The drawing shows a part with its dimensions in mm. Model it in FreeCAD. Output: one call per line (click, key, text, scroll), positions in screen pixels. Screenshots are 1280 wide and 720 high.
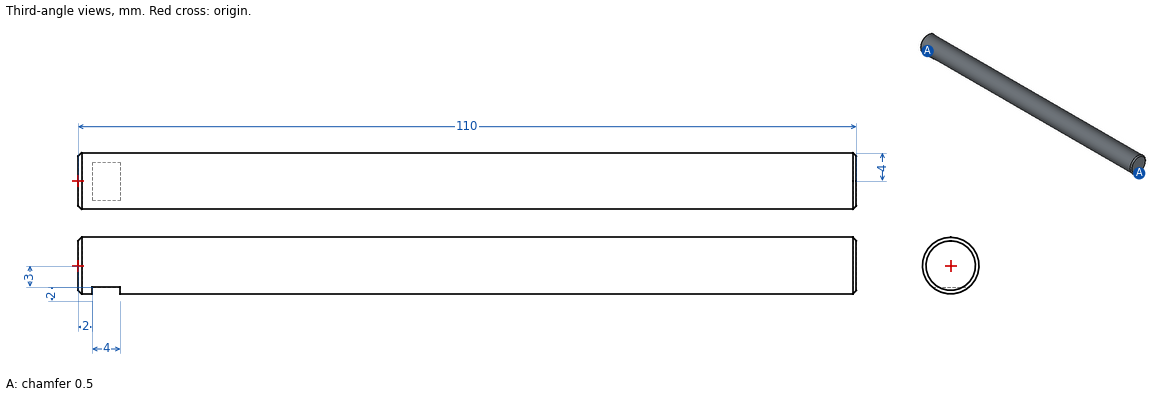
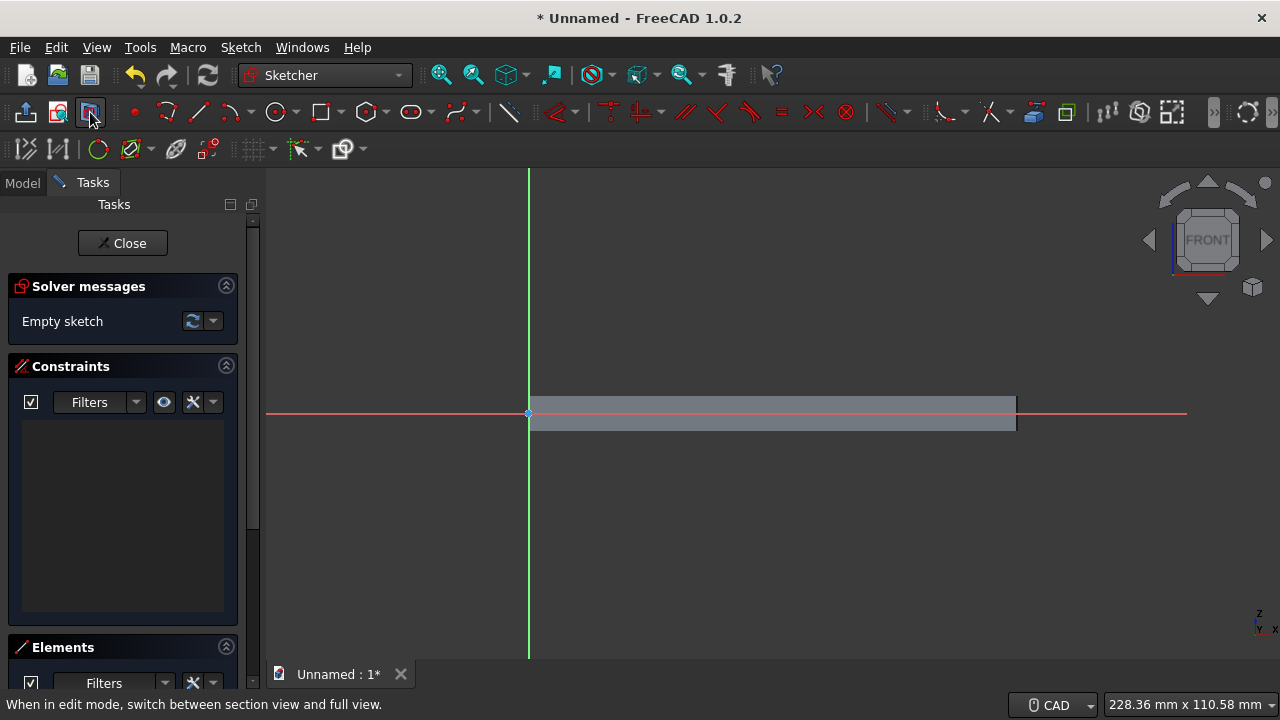
scroll(529, 425, up, 13)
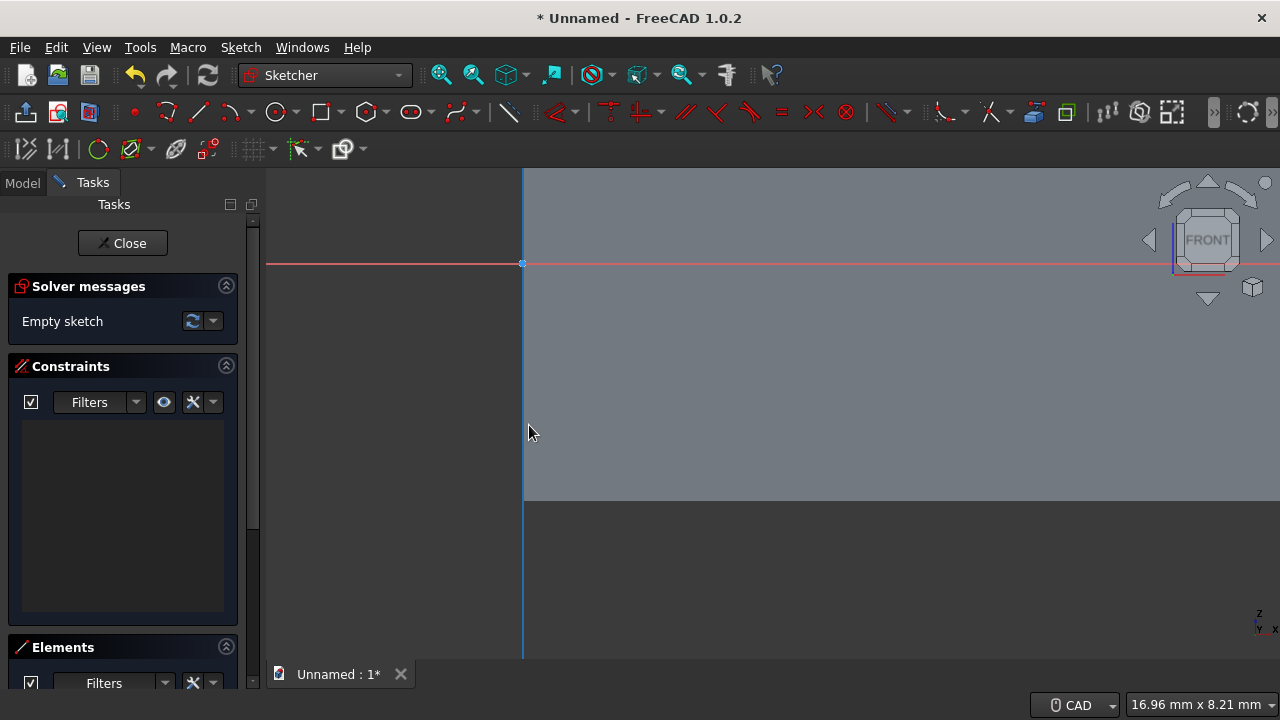
click(322, 112)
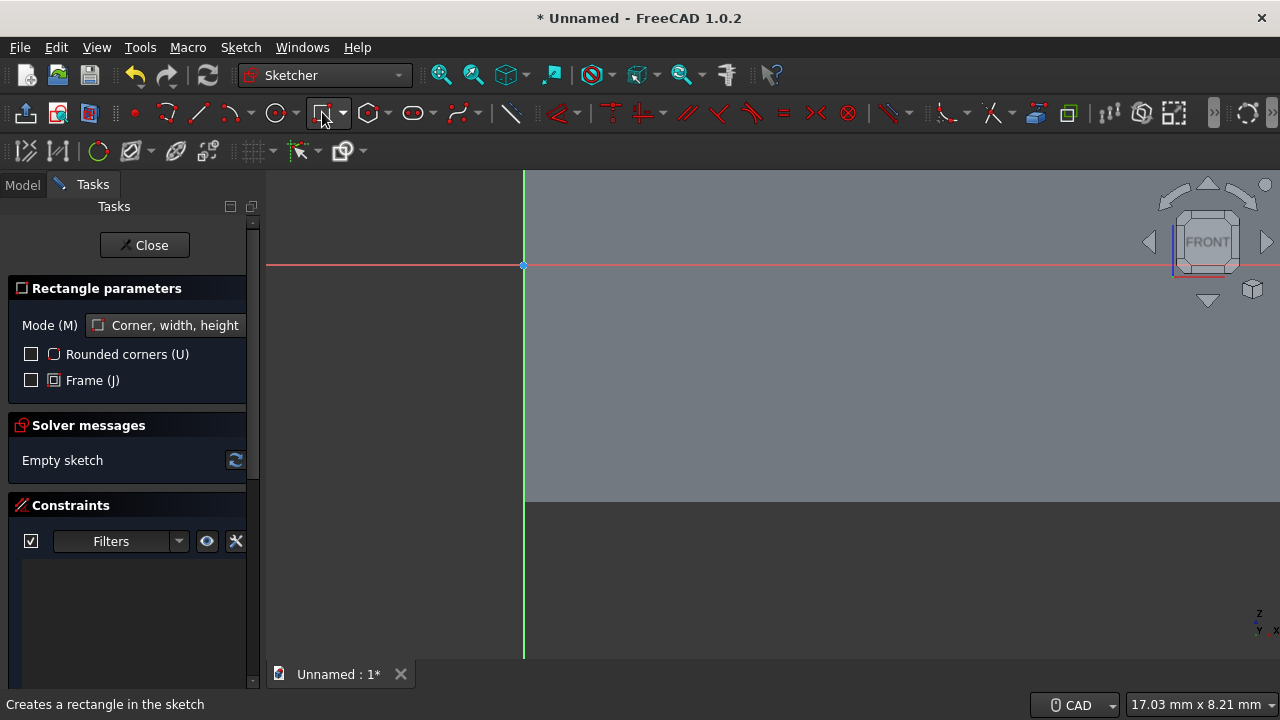
click(643, 444)
click(881, 563)
key(Escape)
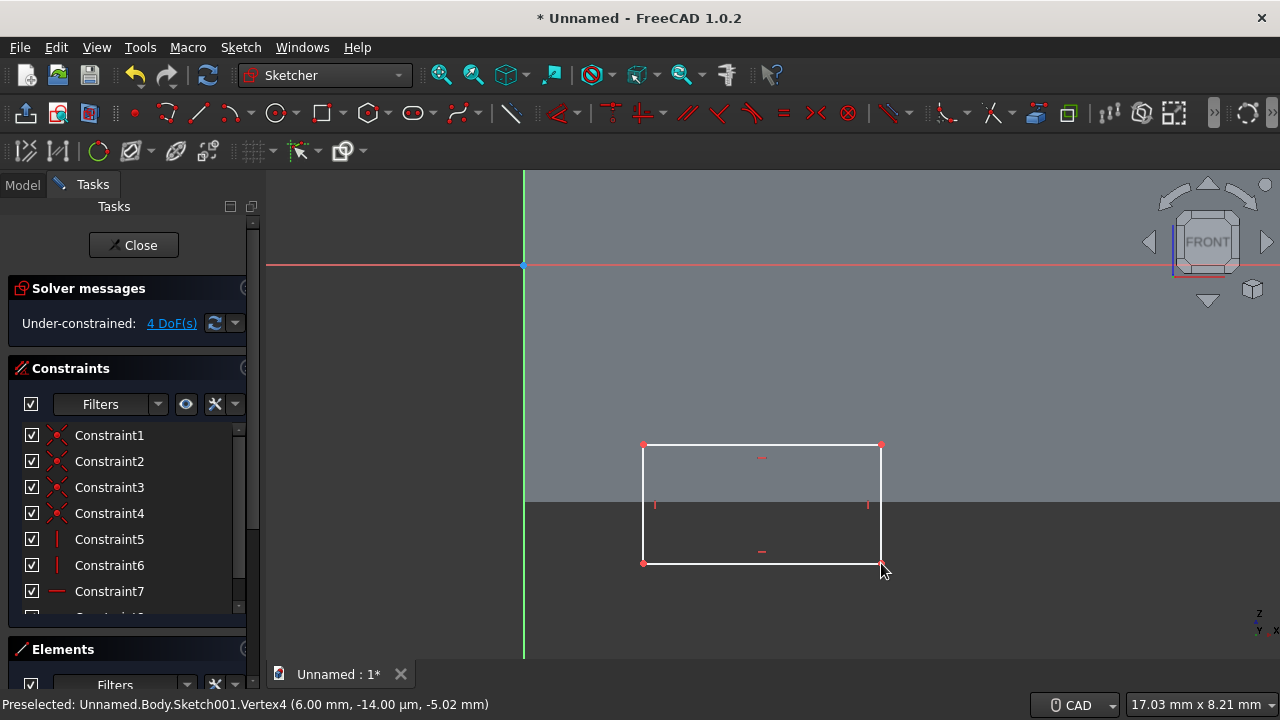
click(558, 114)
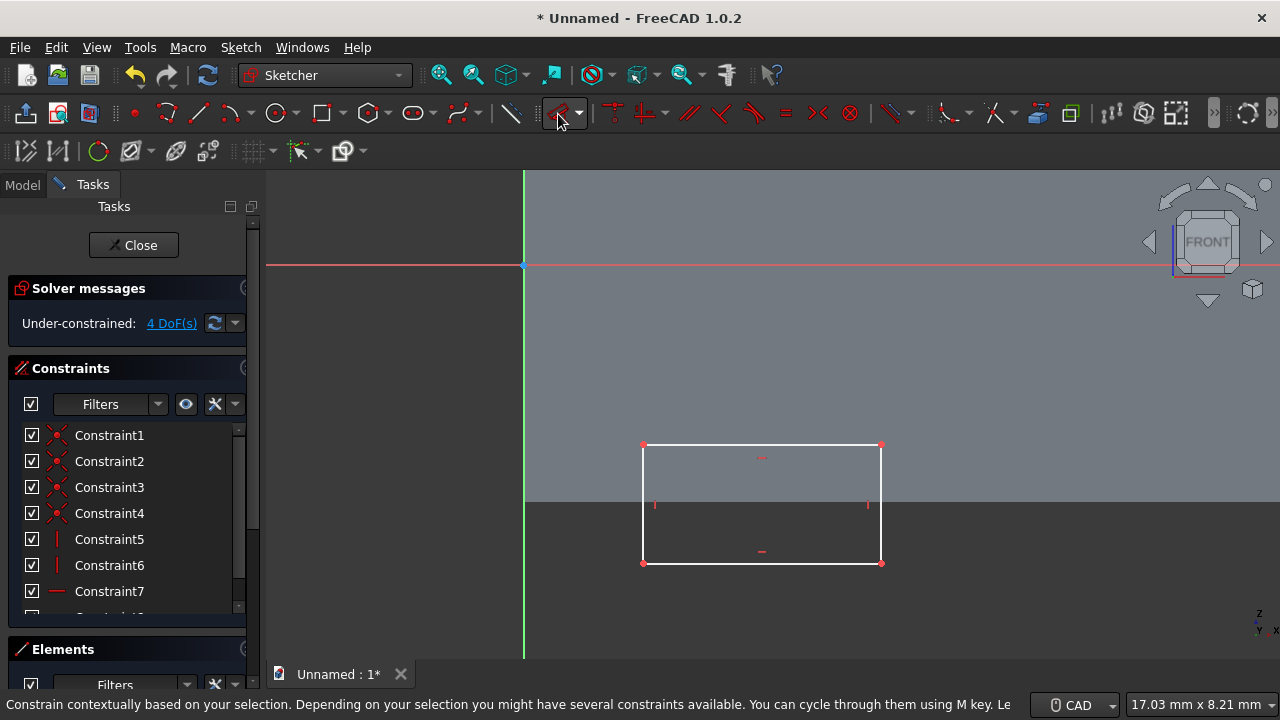
click(643, 481)
click(609, 504)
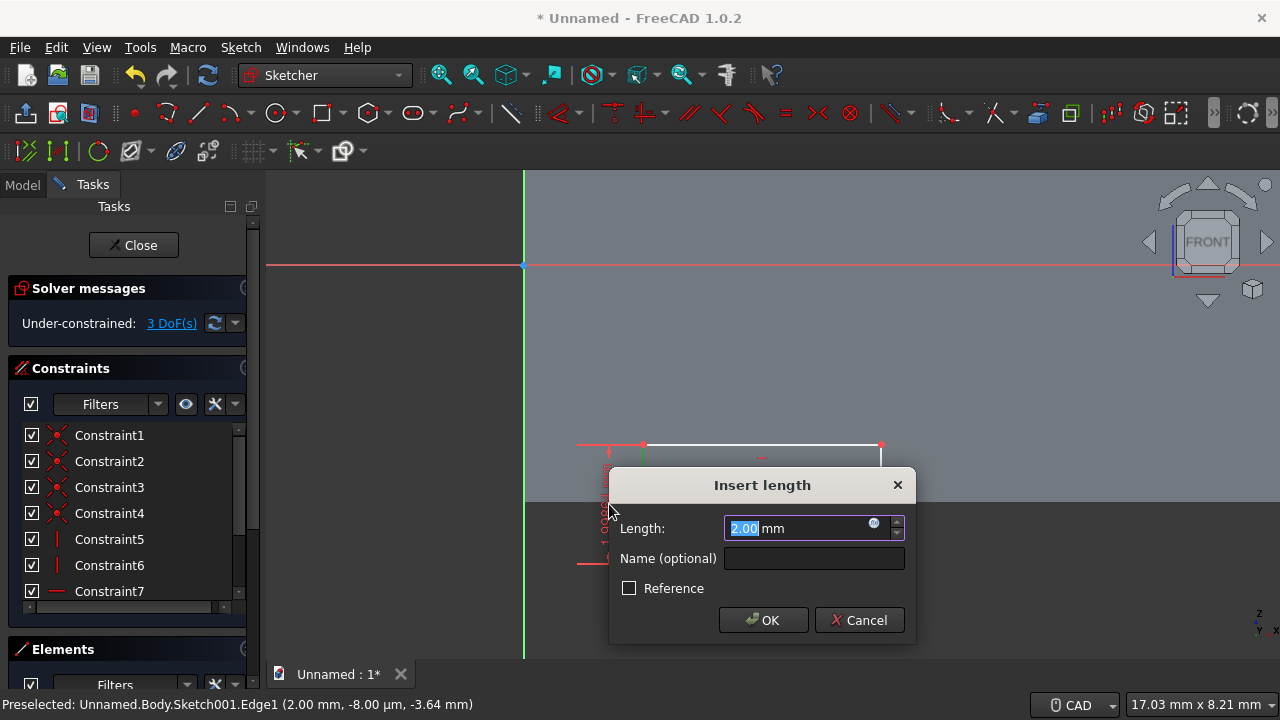
text(2)
key(Return)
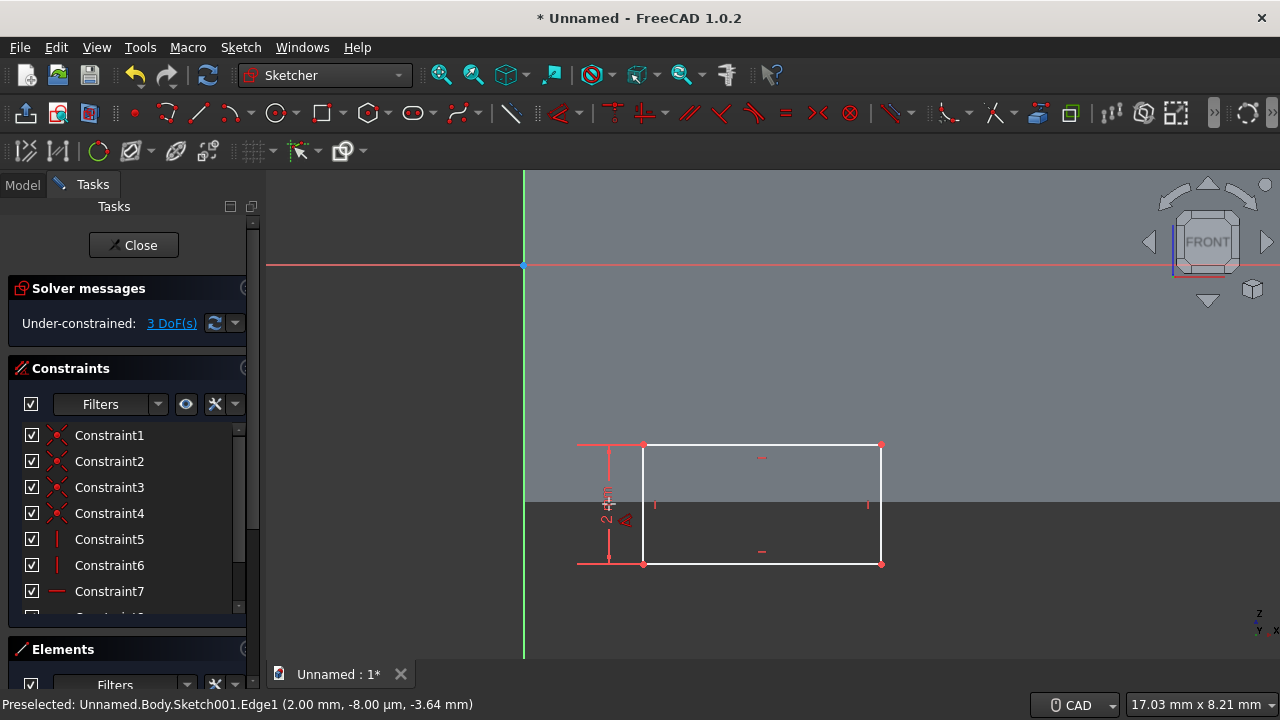
click(714, 564)
click(762, 598)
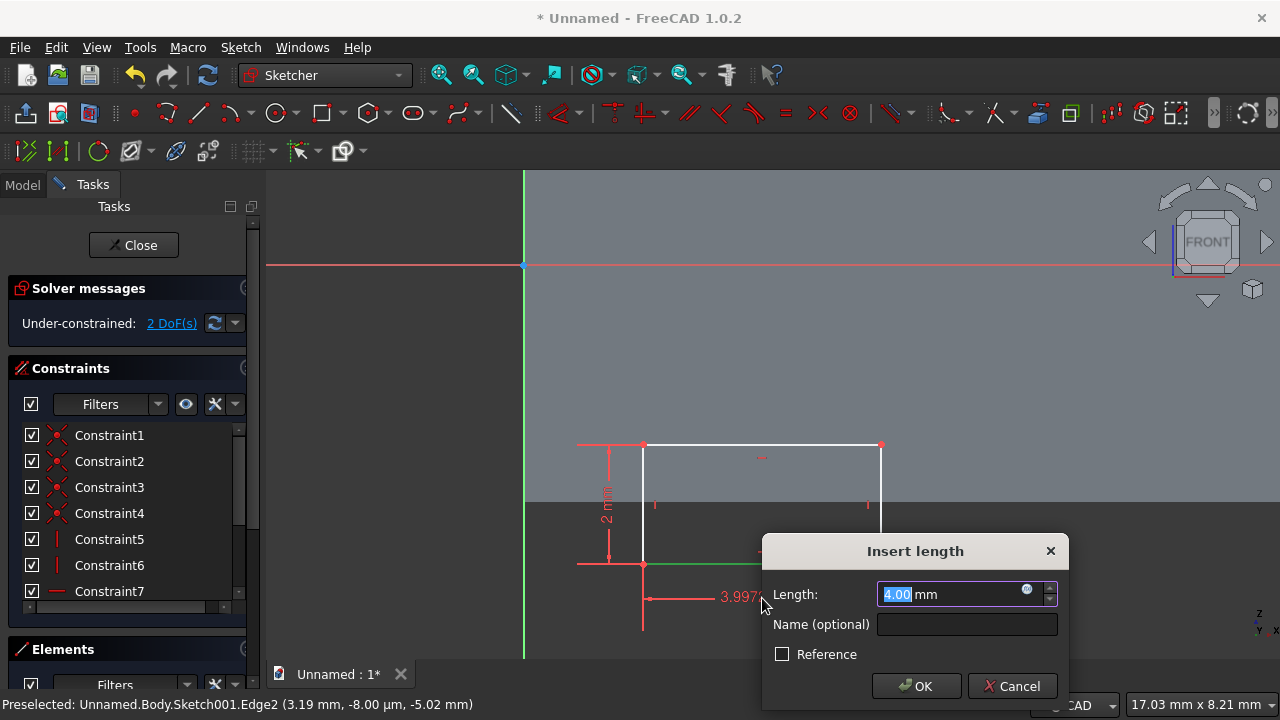
text(4)
key(Return)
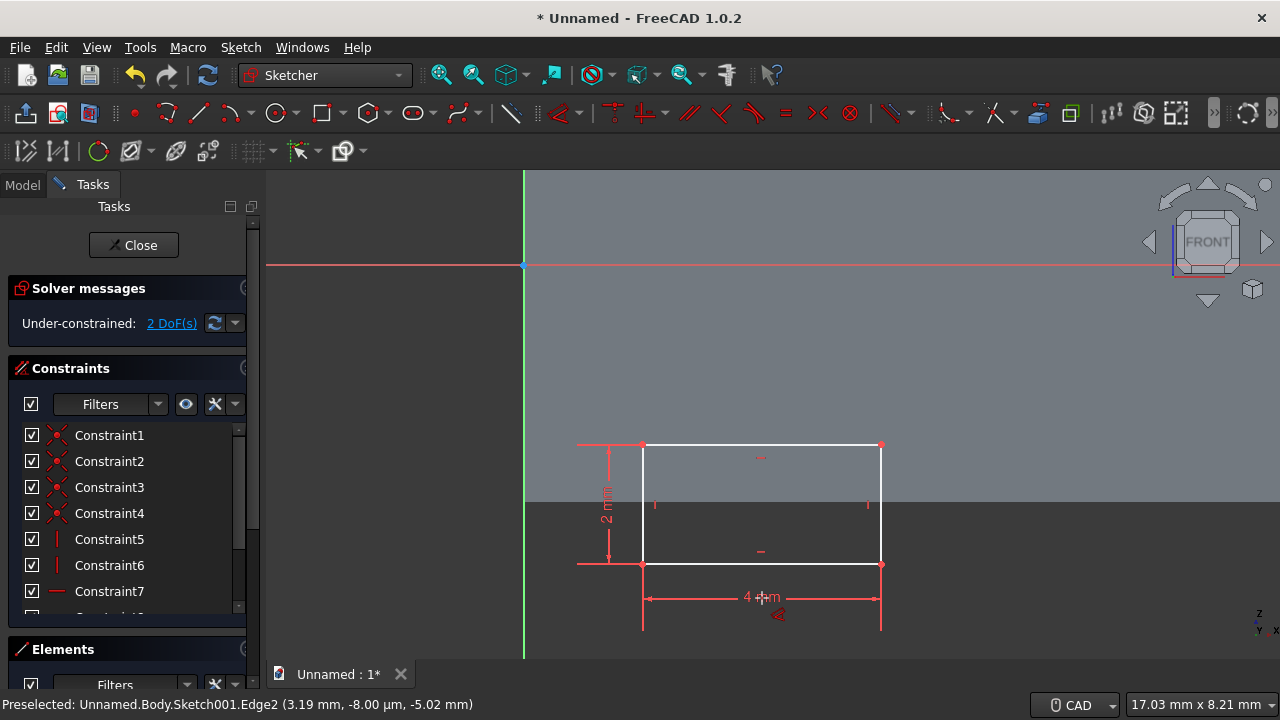
click(643, 445)
click(583, 231)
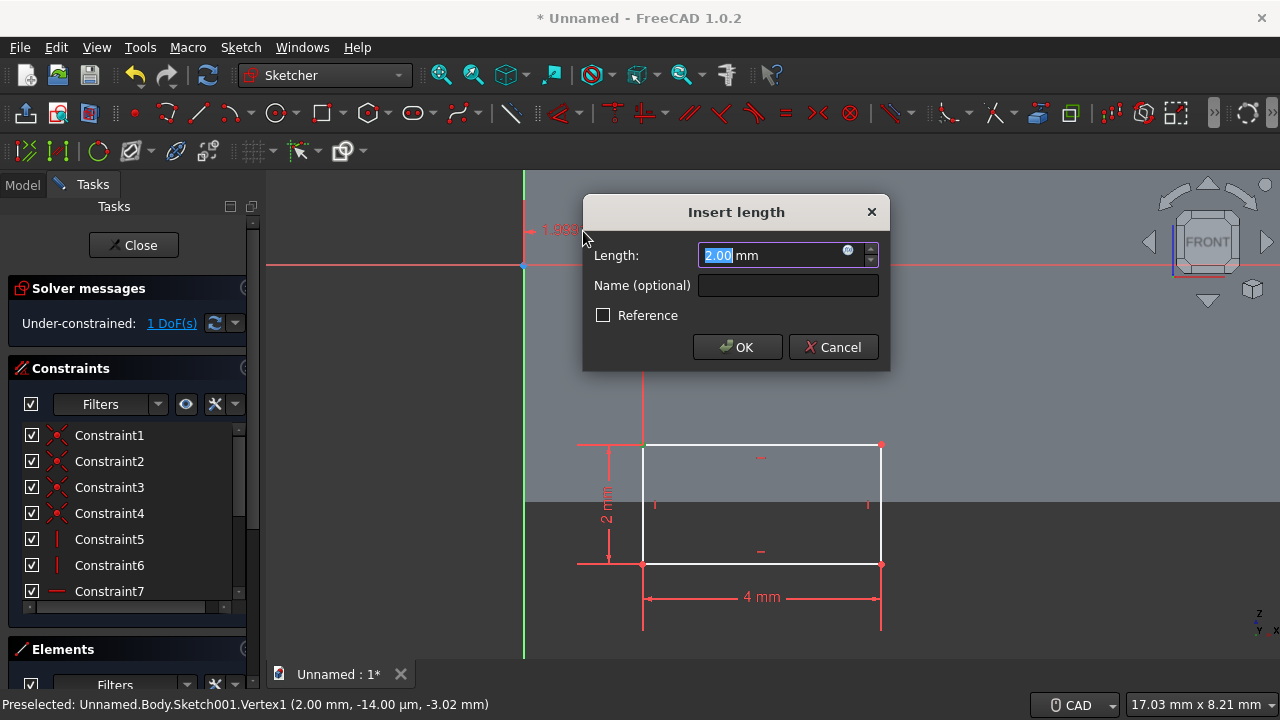
text(2)
key(Return)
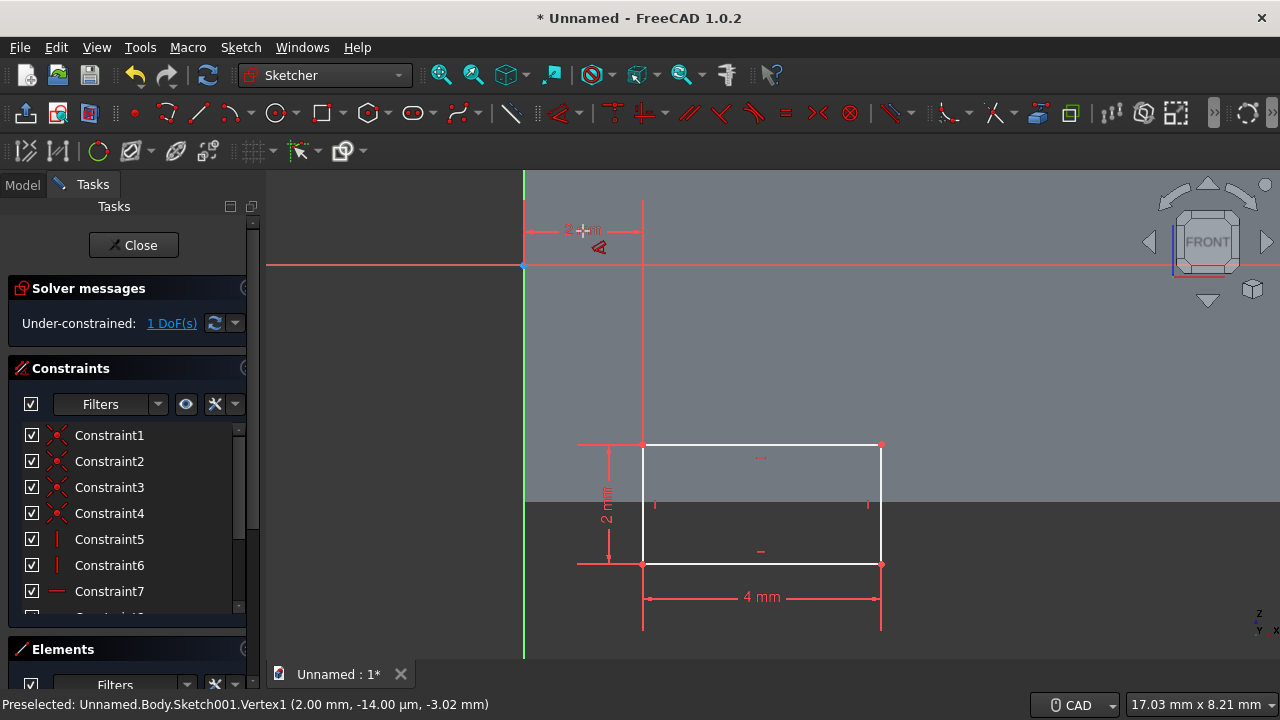
click(643, 445)
click(490, 355)